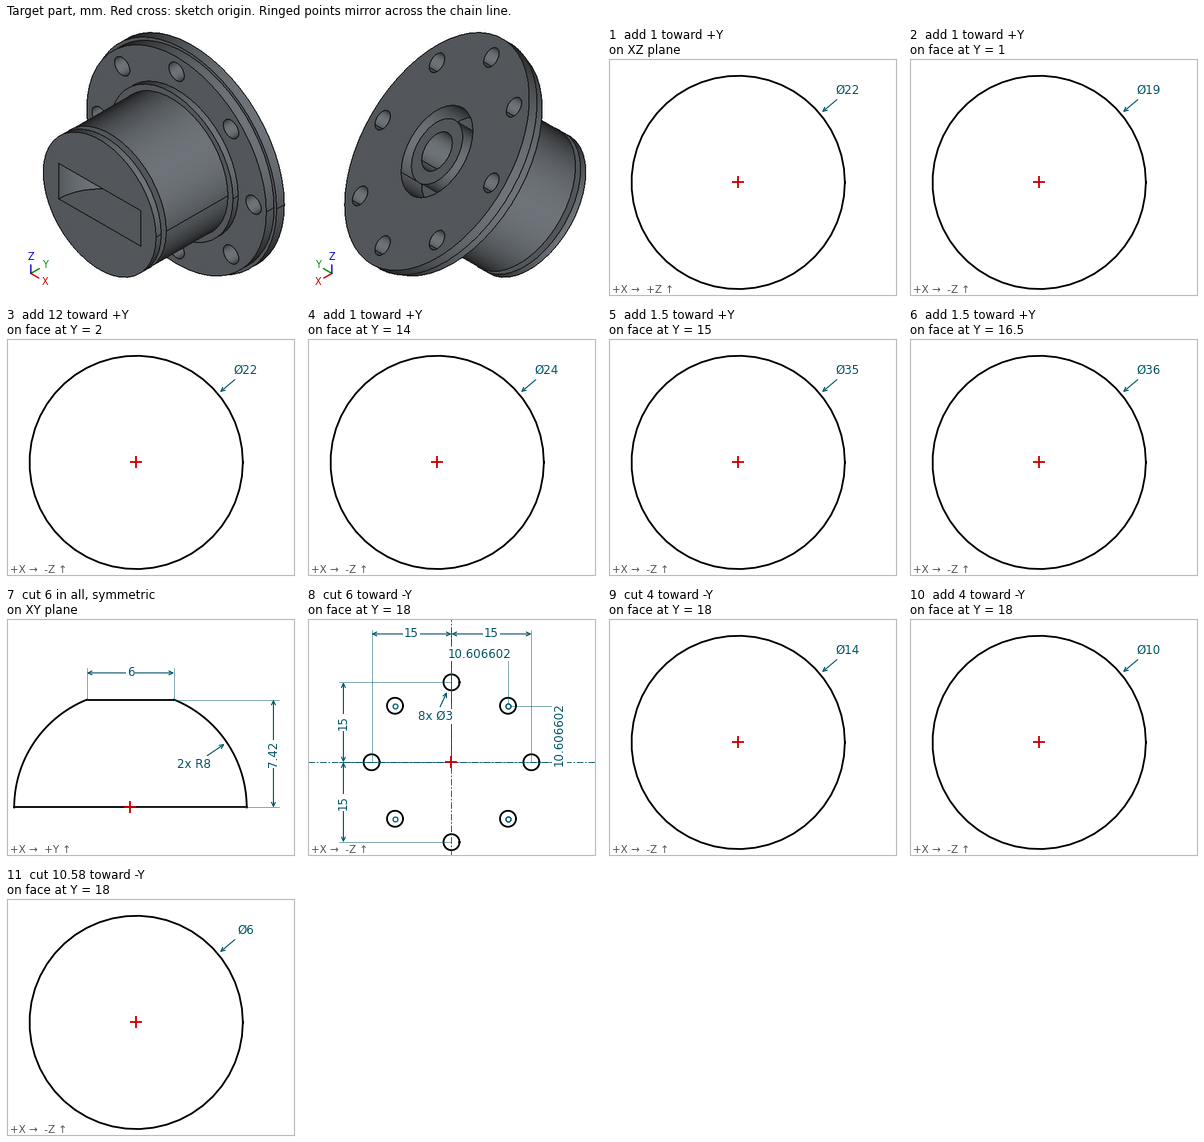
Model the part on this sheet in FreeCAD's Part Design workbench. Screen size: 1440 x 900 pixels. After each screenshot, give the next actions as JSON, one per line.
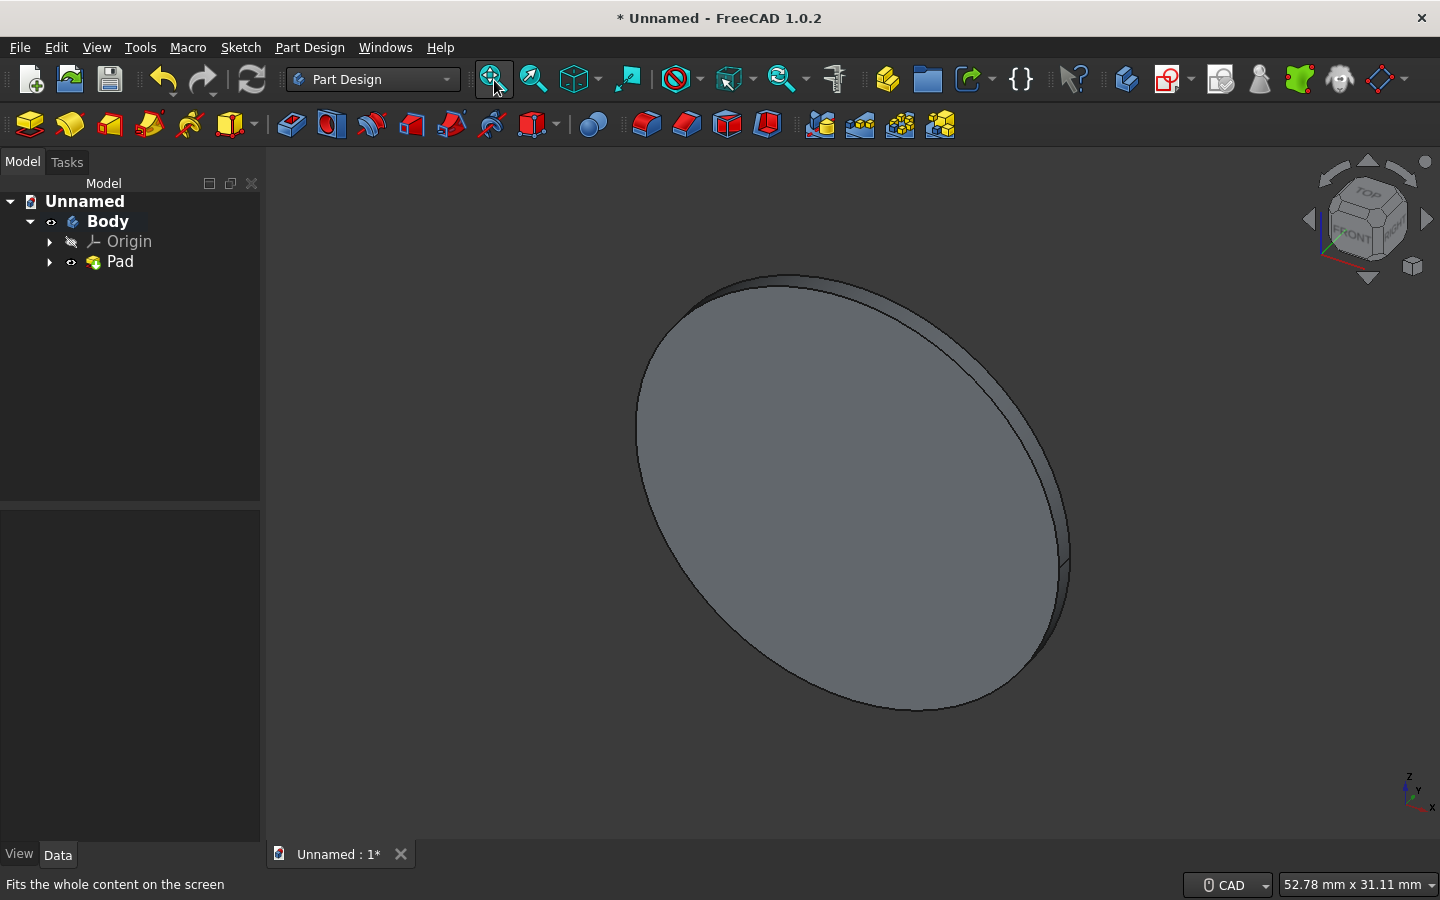
{"action": "key", "text": "4"}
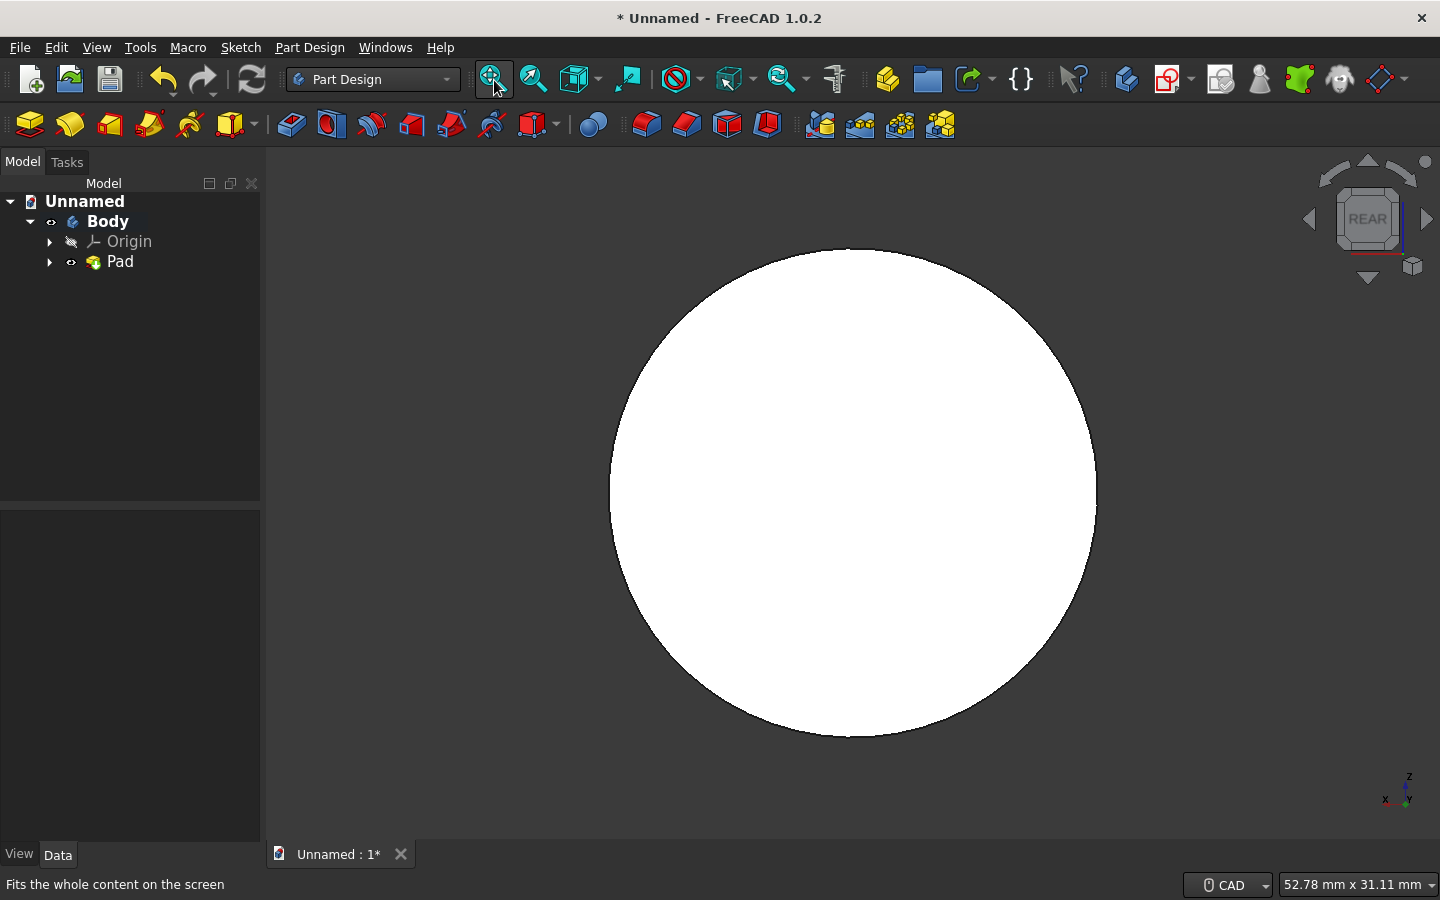
{"action": "left_click", "coordinate": [853, 492]}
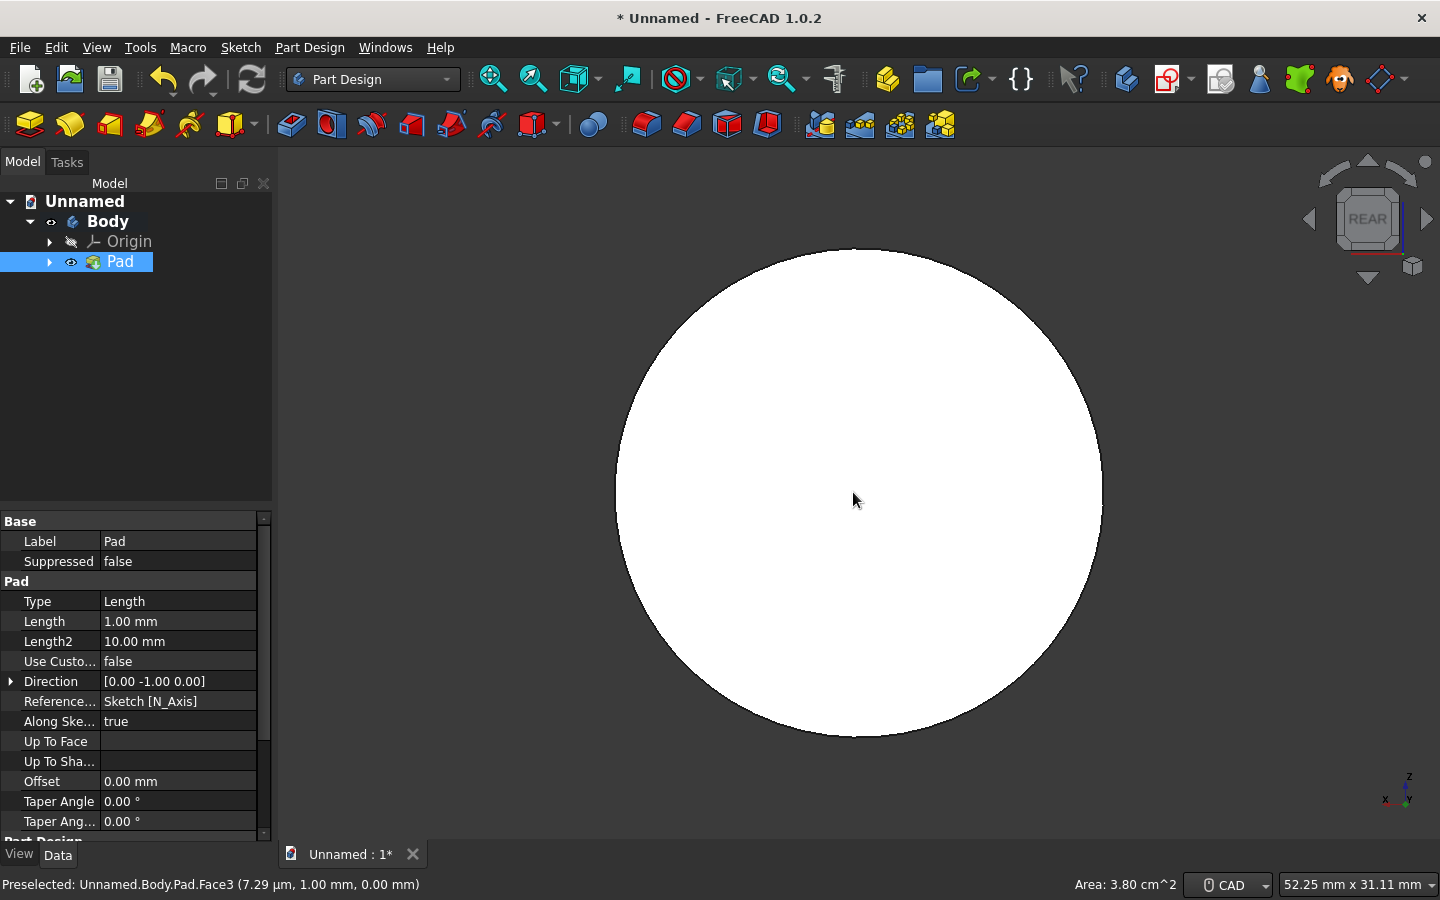
{"action": "left_click", "coordinate": [1168, 80]}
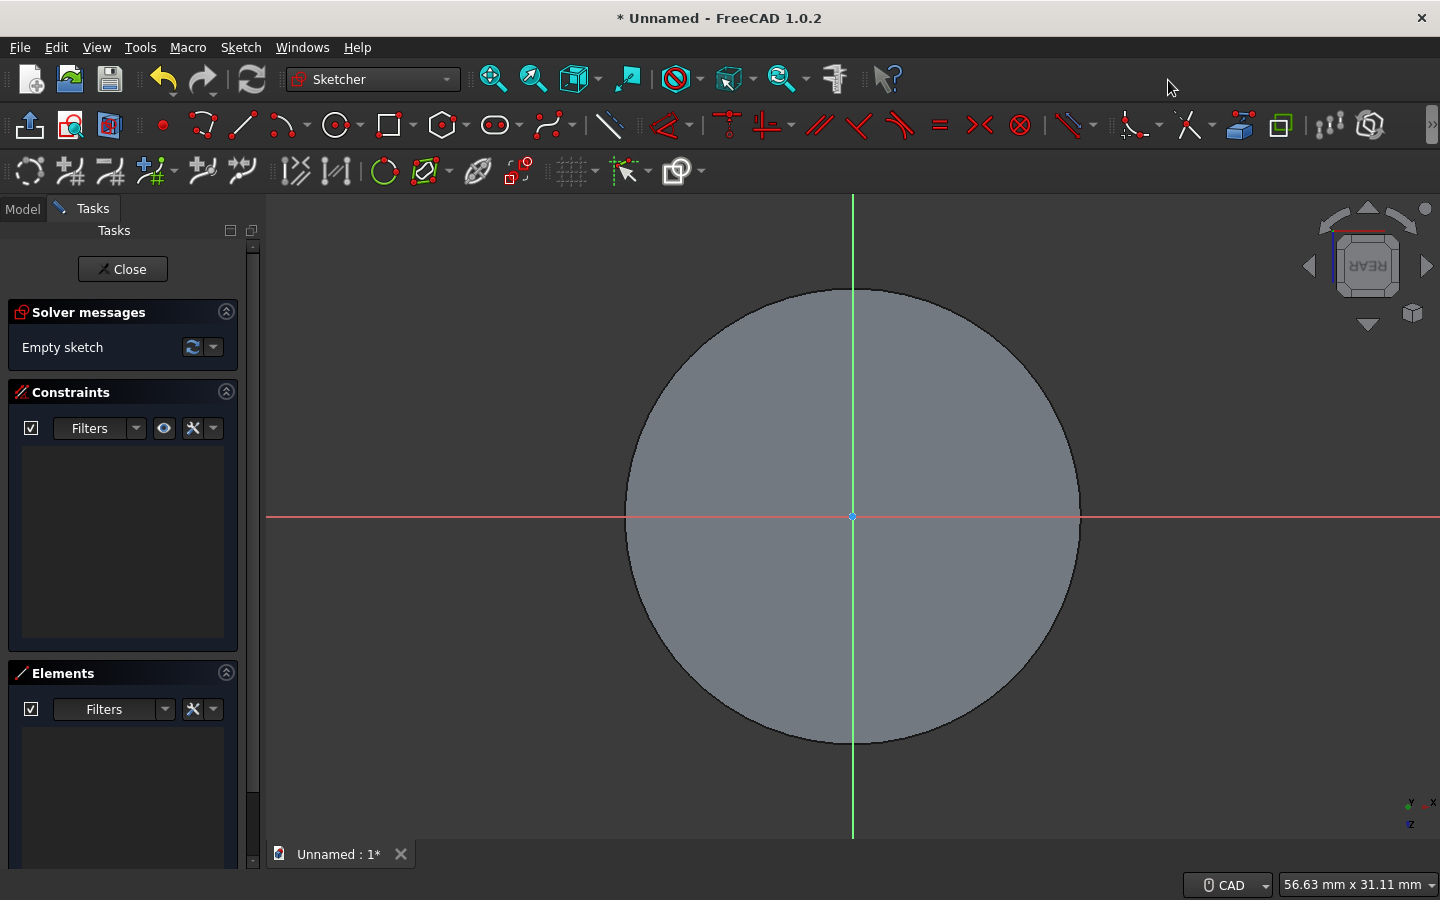
{"action": "left_click", "coordinate": [336, 126]}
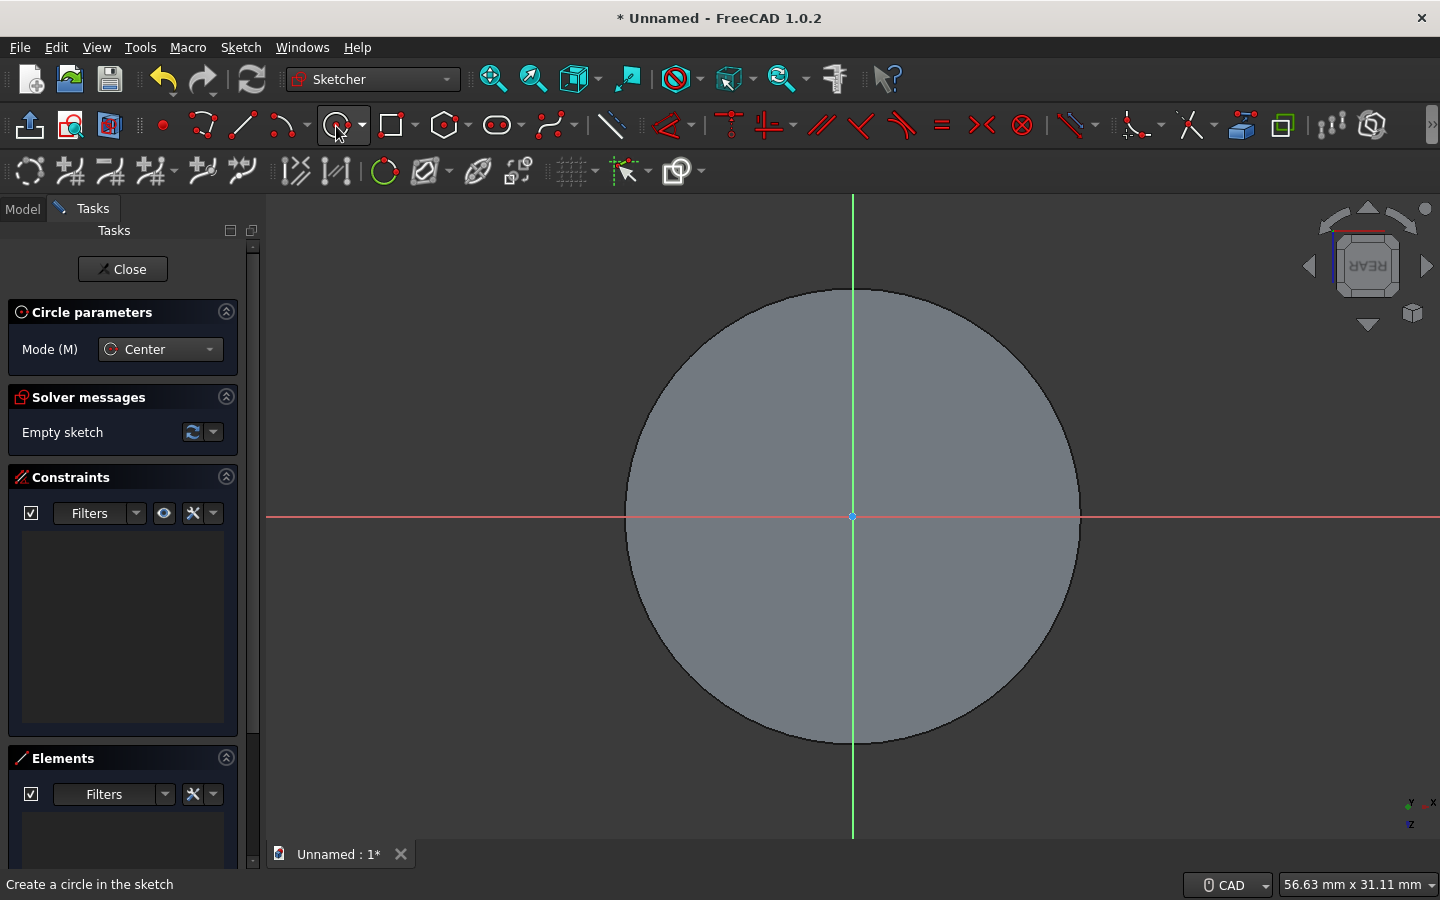
{"action": "left_click", "coordinate": [853, 516]}
{"action": "mouse_move", "coordinate": [992, 377]}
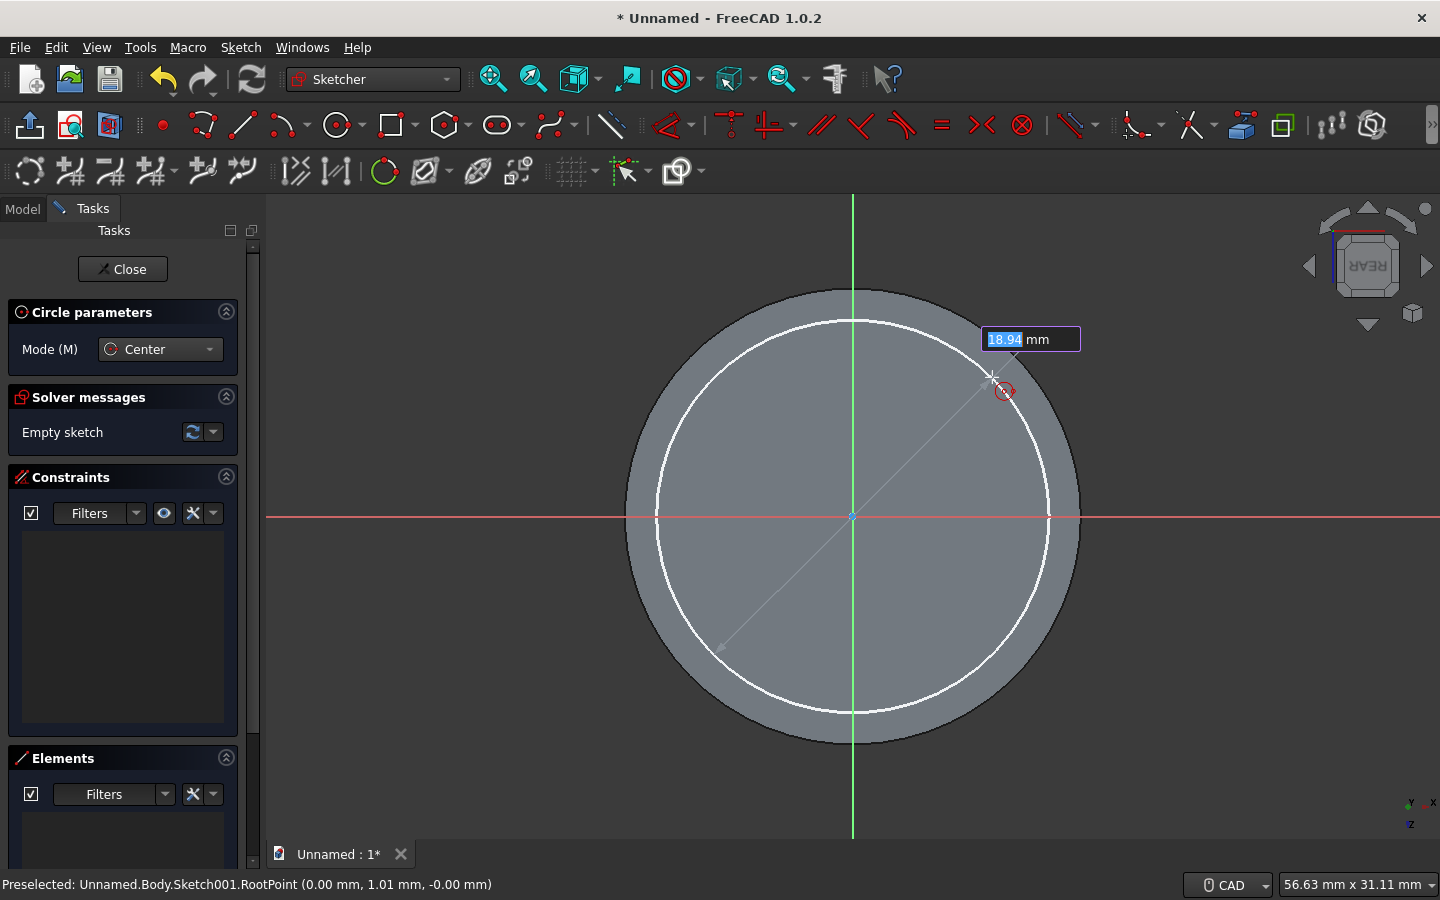
{"action": "type", "text": "19"}
{"action": "key", "text": "Return"}
{"action": "key", "text": "Escape"}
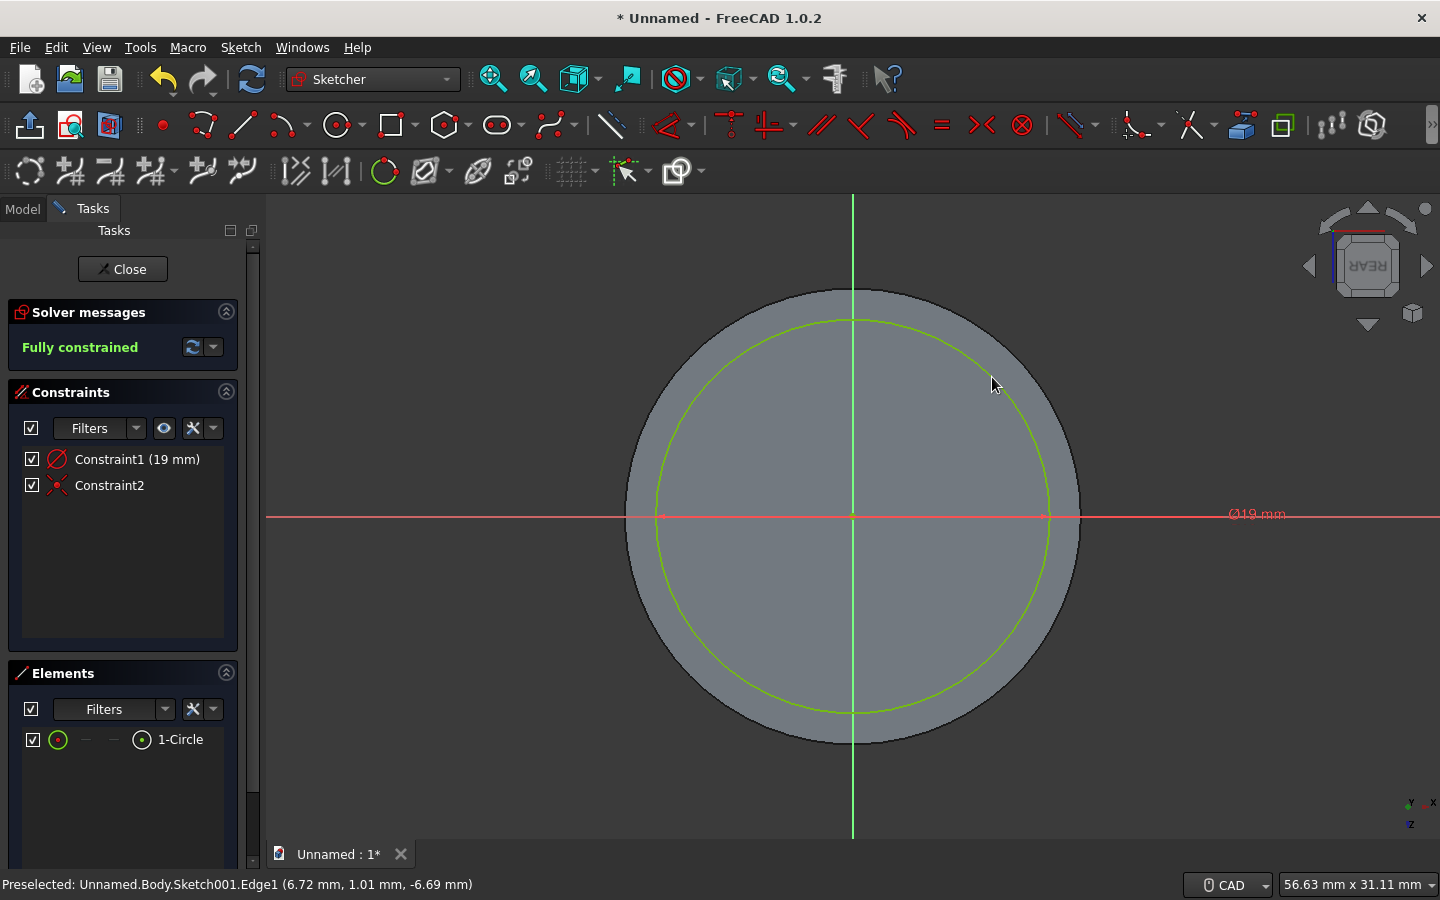
{"action": "left_click", "coordinate": [123, 269]}